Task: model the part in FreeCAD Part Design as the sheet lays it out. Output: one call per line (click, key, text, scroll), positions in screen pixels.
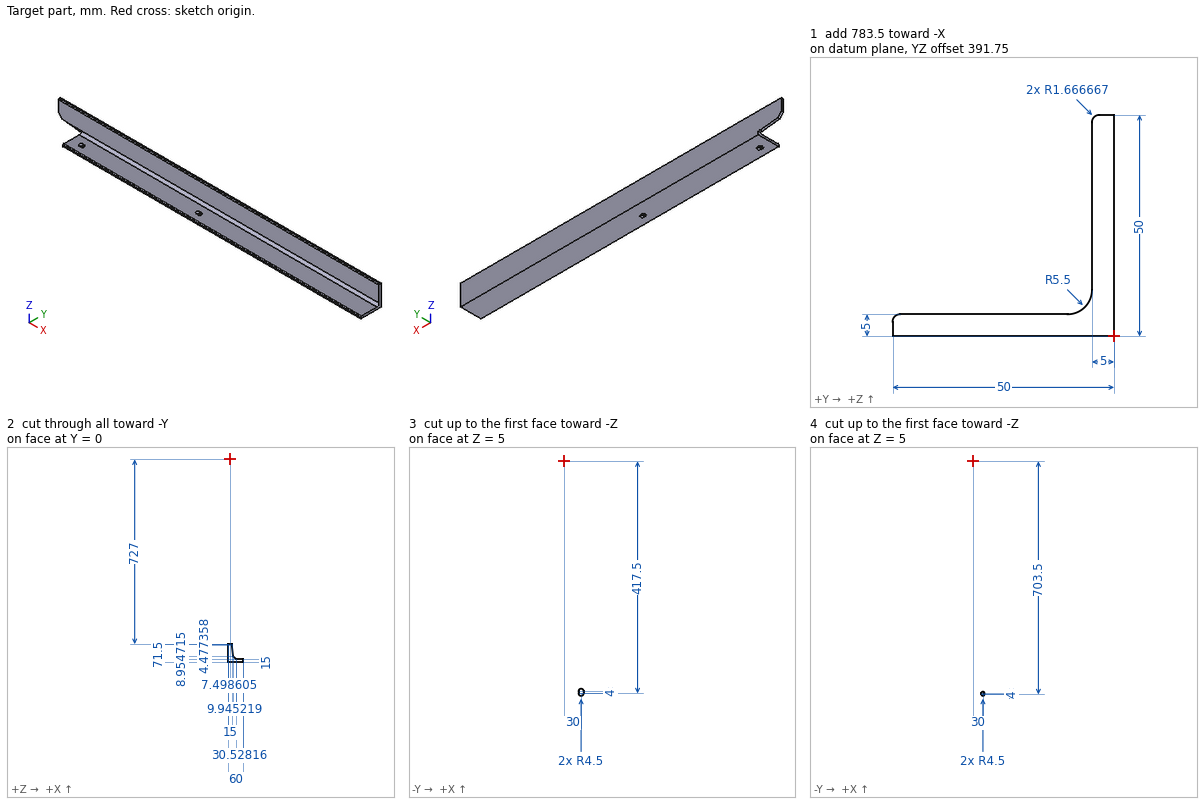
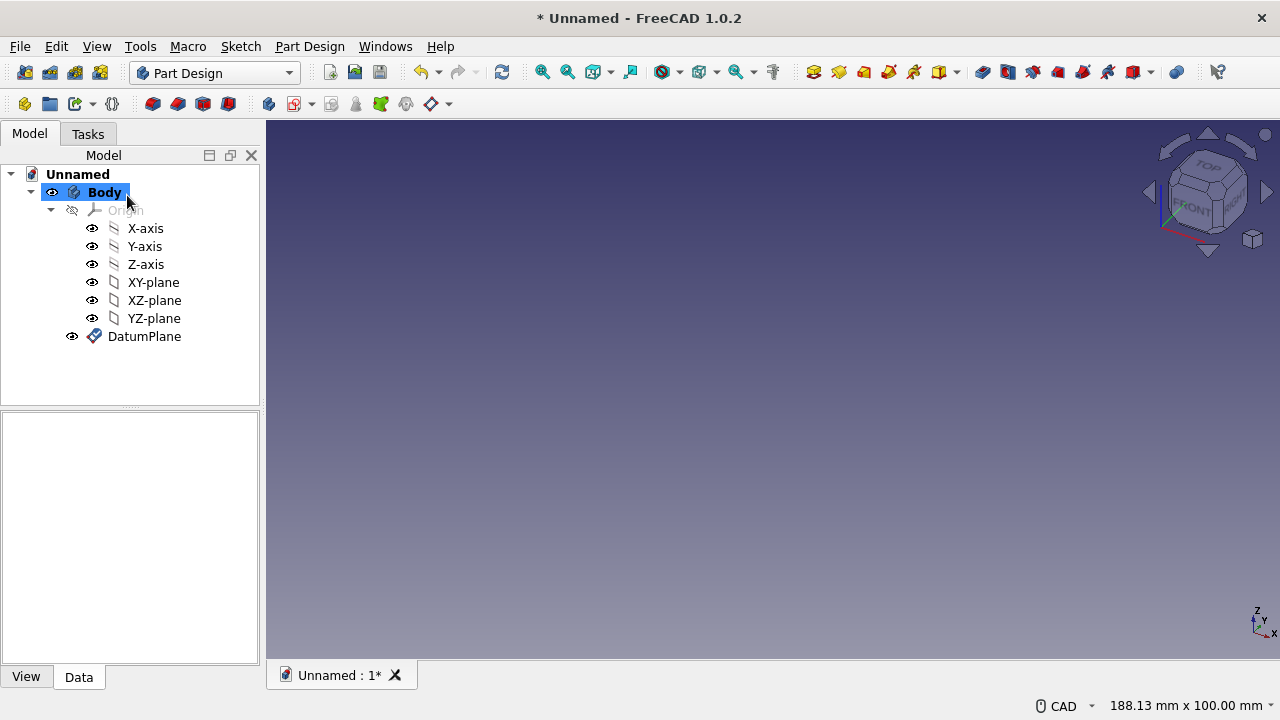
click(117, 336)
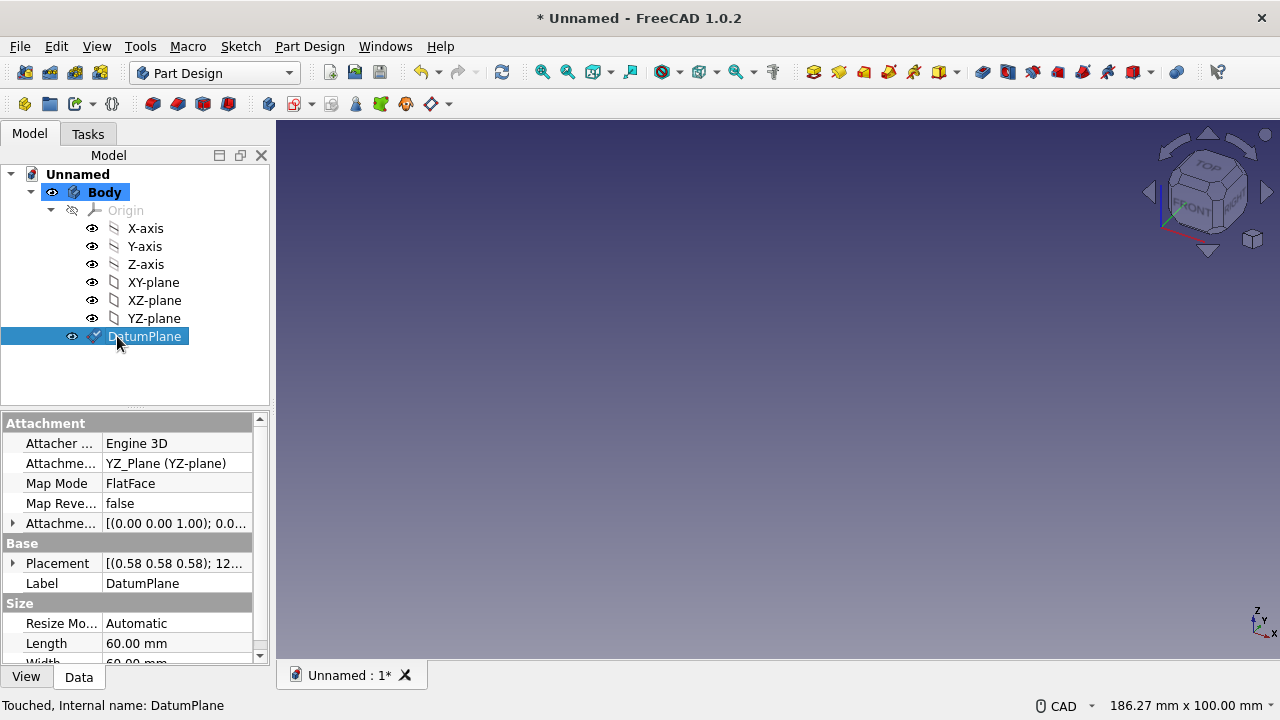
click(294, 104)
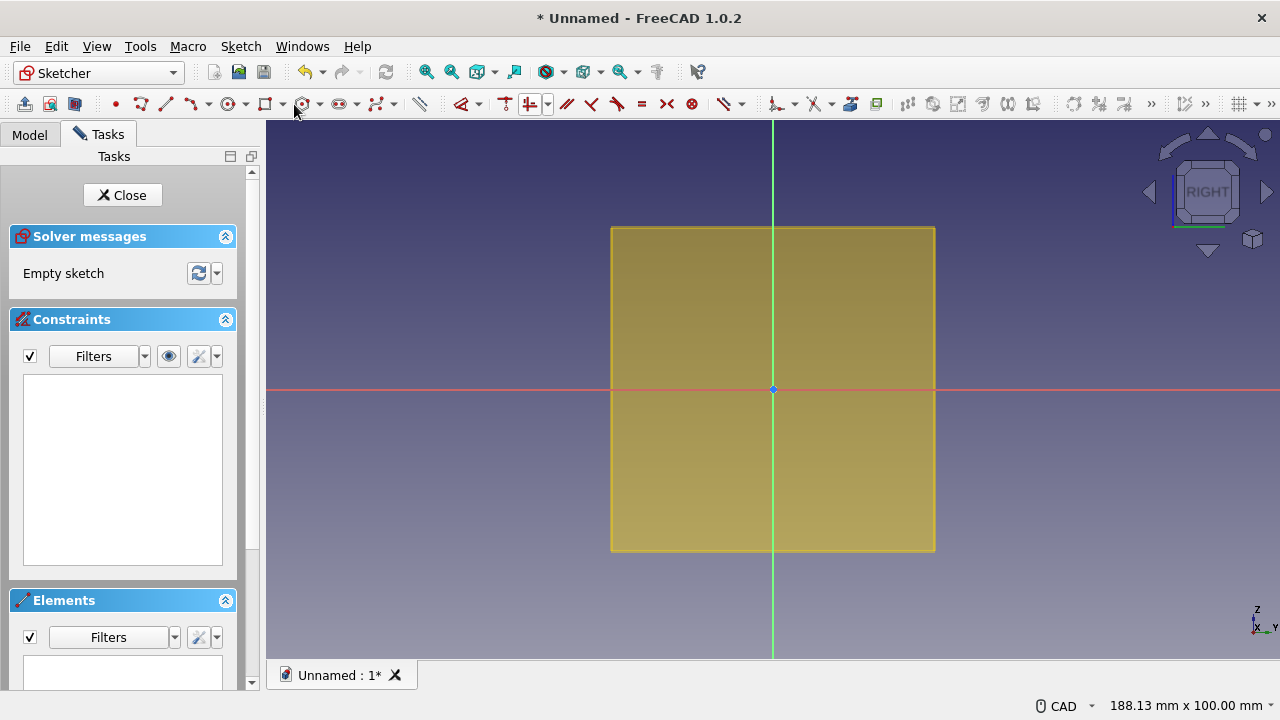
scroll(1004, 631, down, 1)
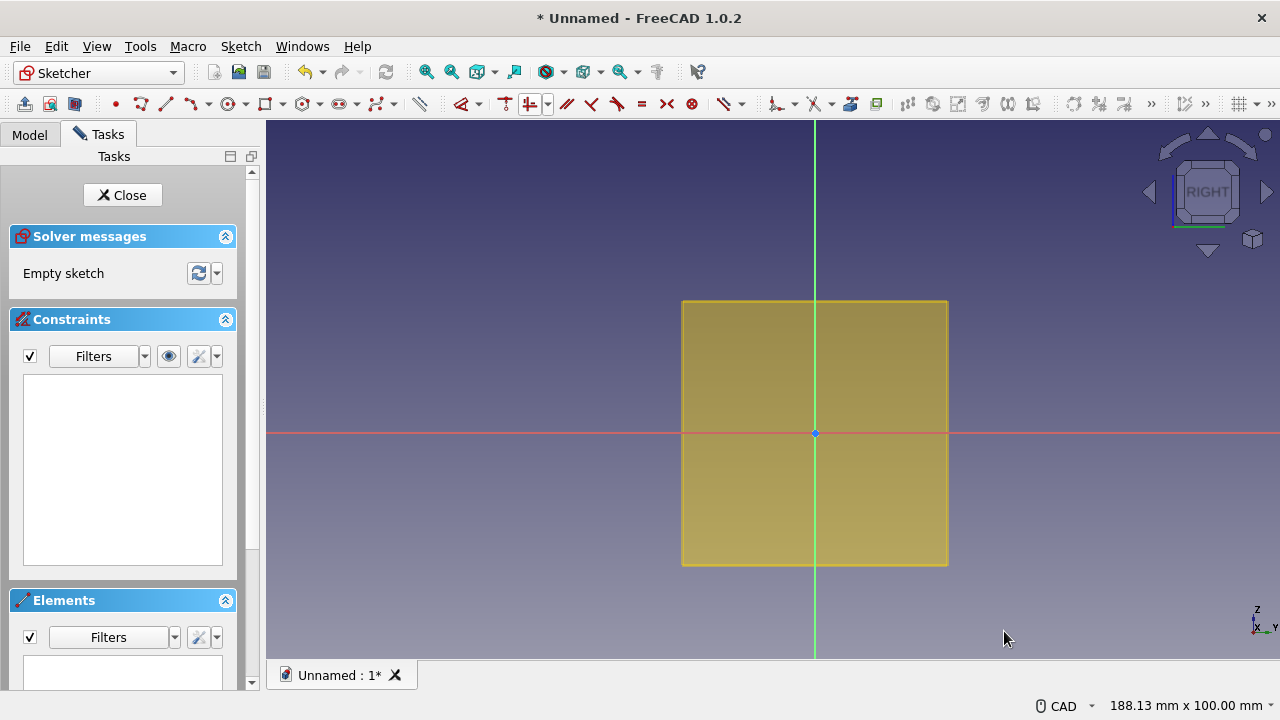
scroll(705, 188, up, 2)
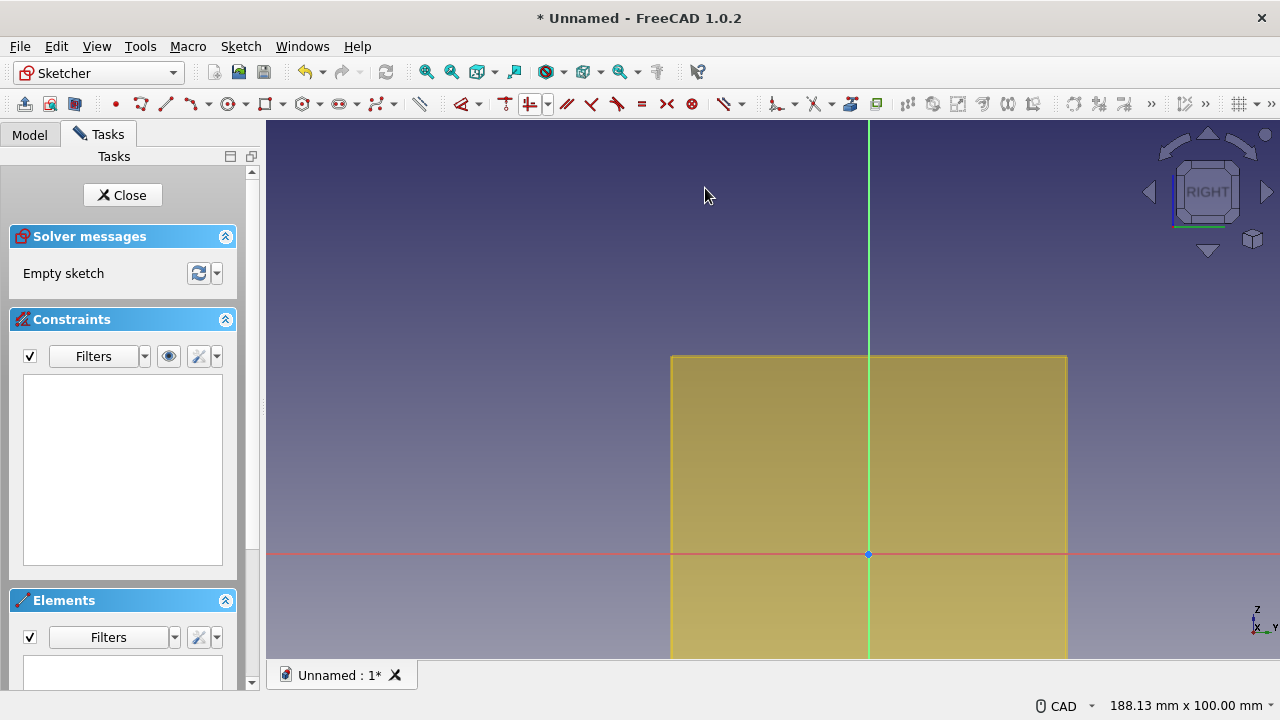
click(166, 104)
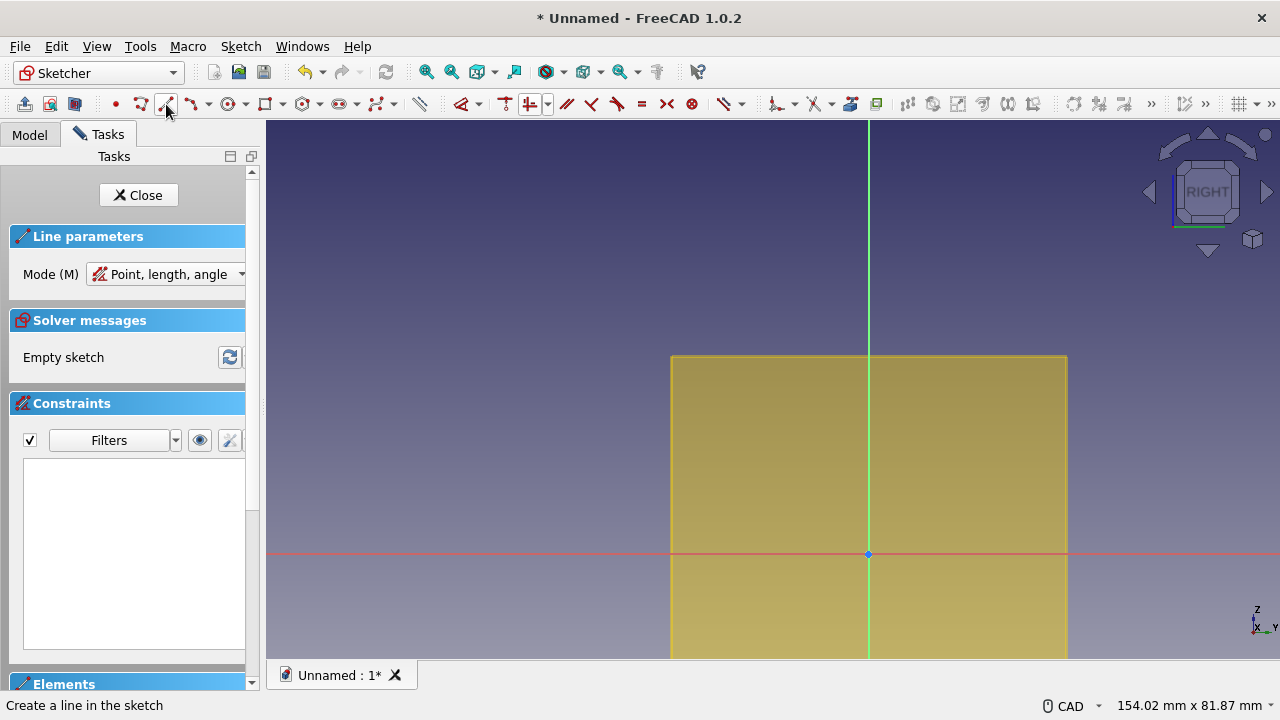
click(551, 521)
click(800, 521)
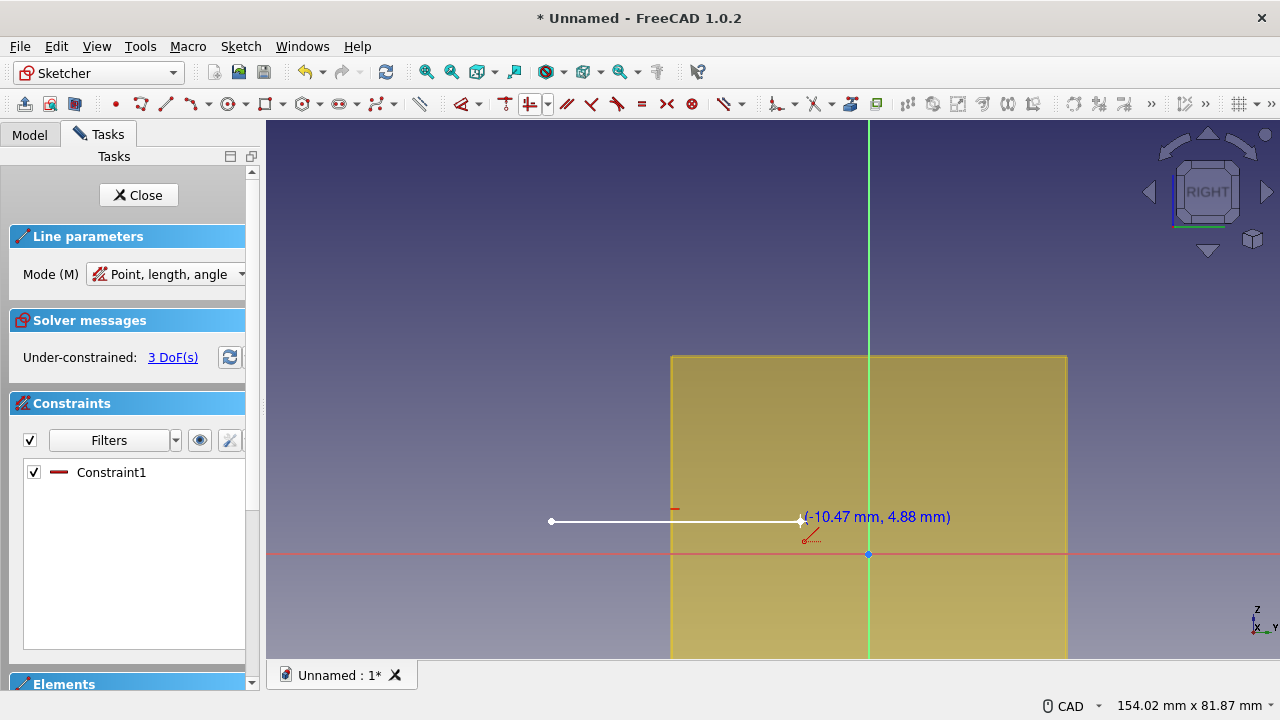
click(836, 485)
click(836, 236)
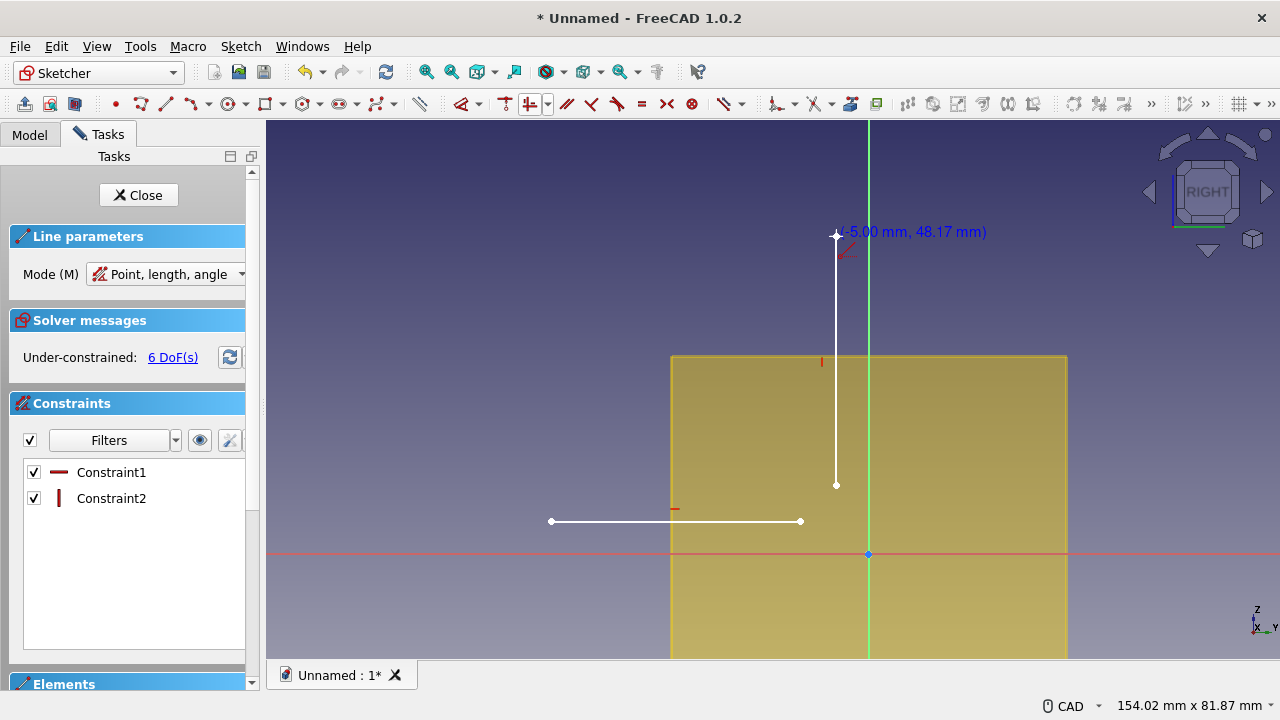
click(141, 104)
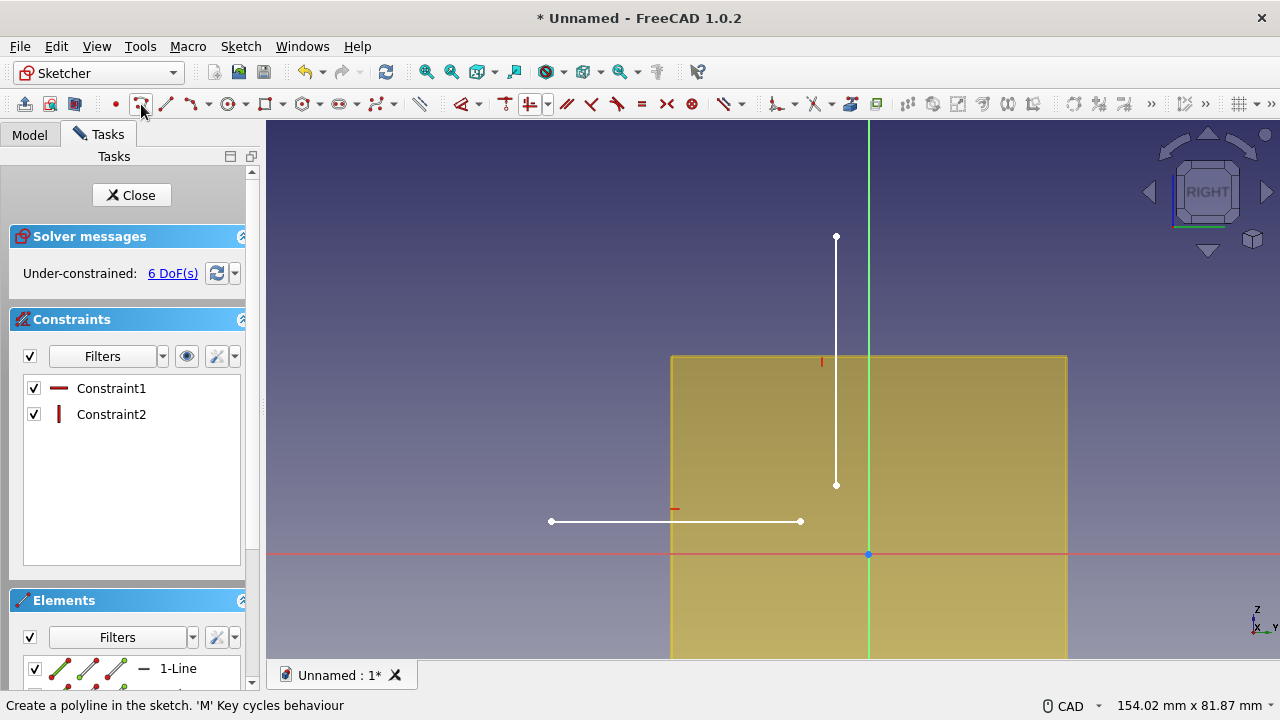
click(847, 225)
click(869, 225)
click(869, 554)
click(540, 545)
click(540, 532)
right_click(540, 532)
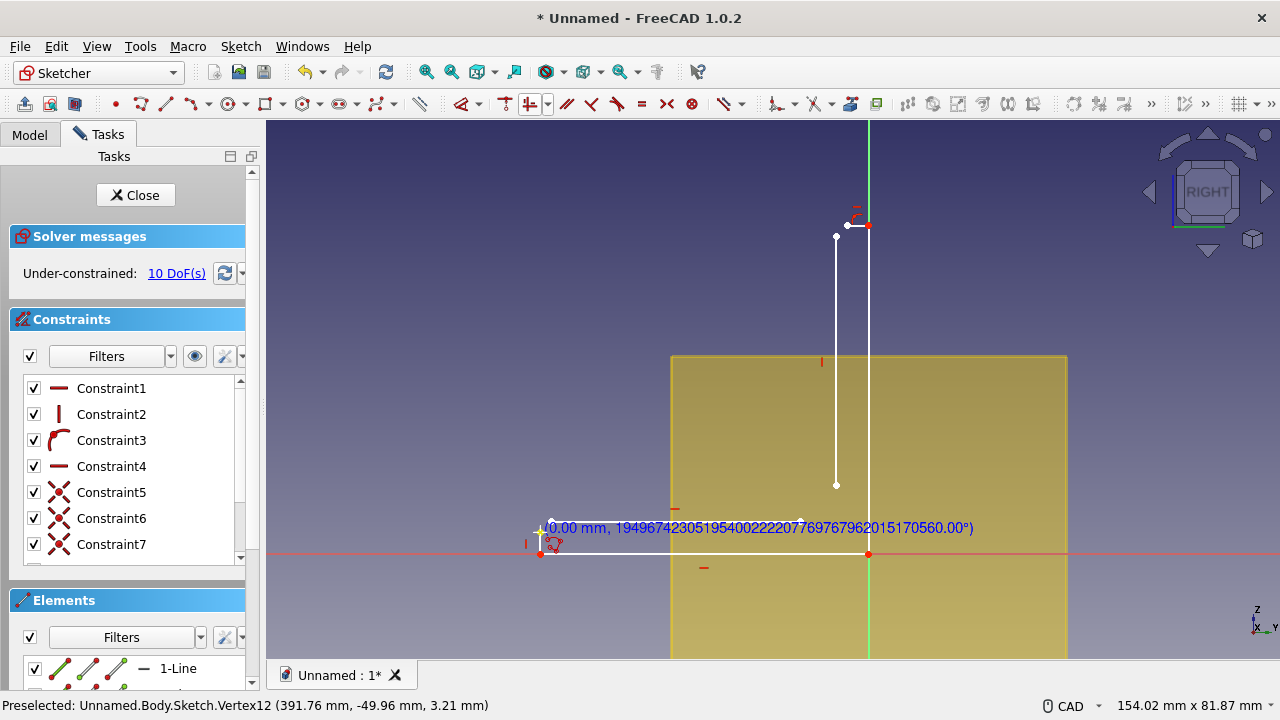
key(g)
key(3)
key(a)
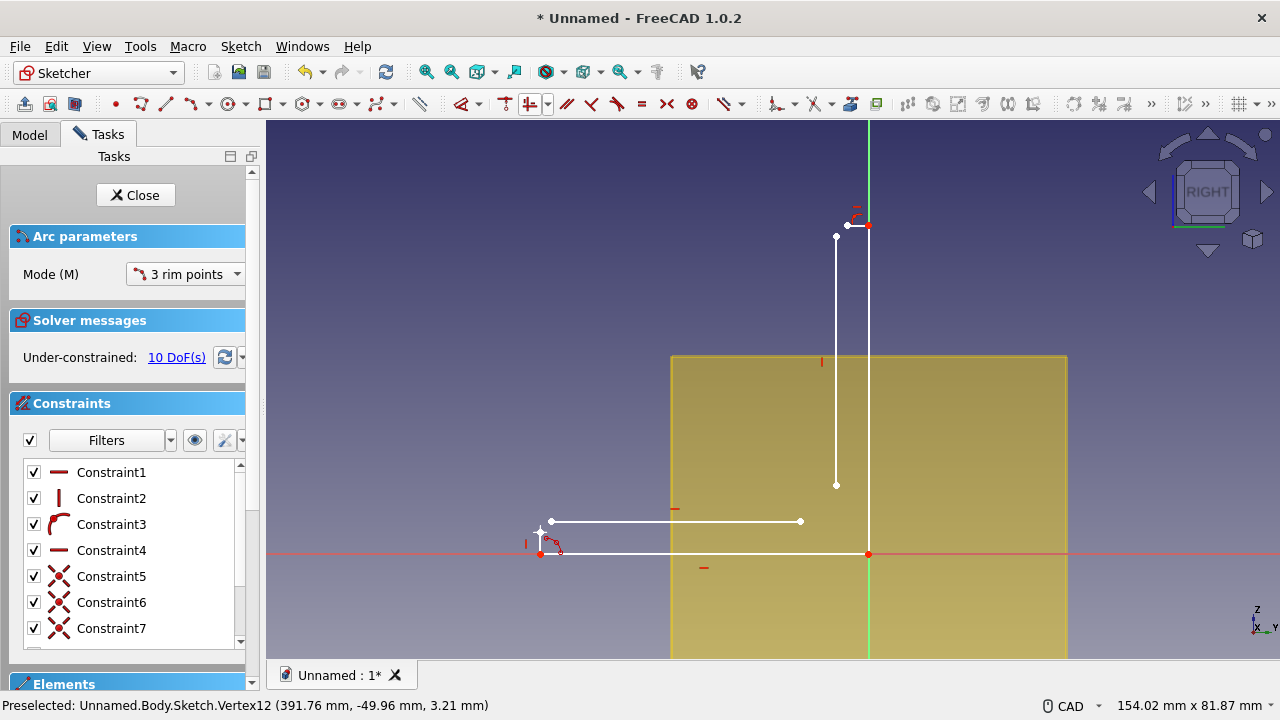
click(800, 522)
click(836, 486)